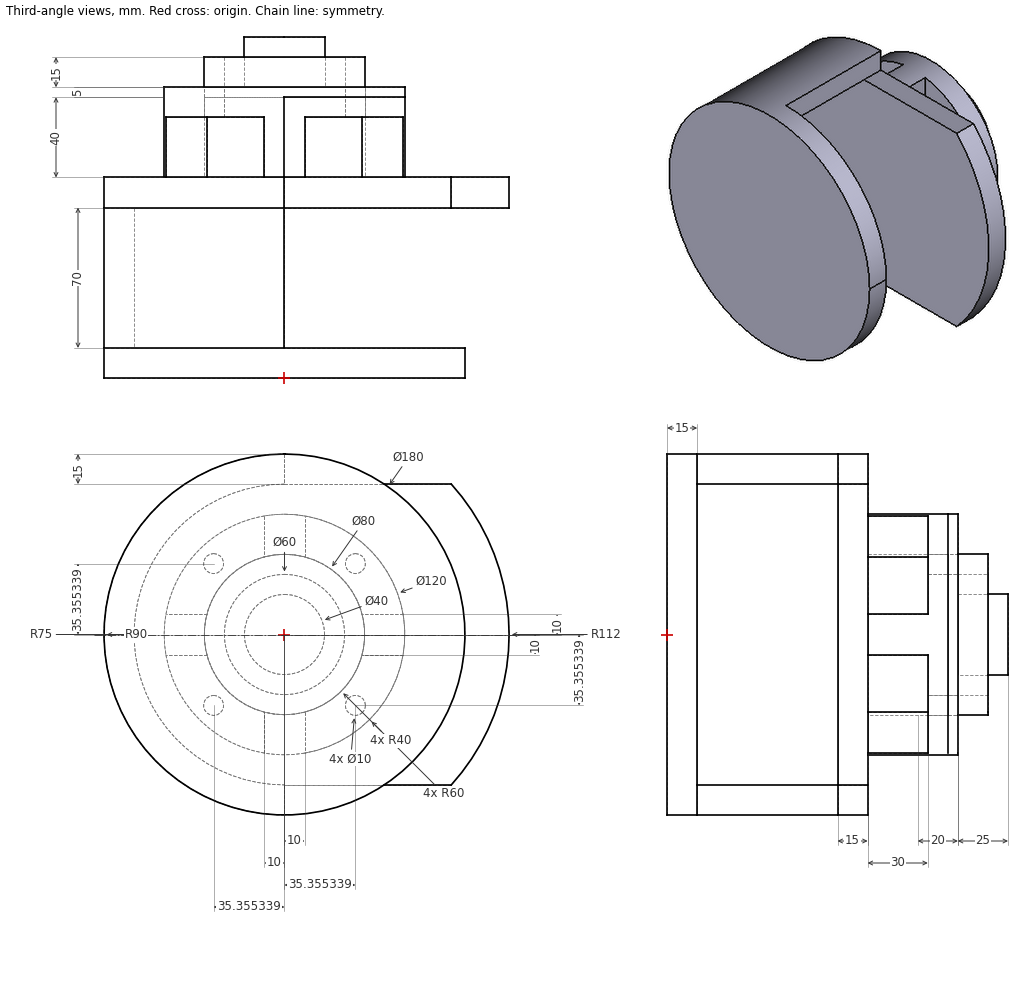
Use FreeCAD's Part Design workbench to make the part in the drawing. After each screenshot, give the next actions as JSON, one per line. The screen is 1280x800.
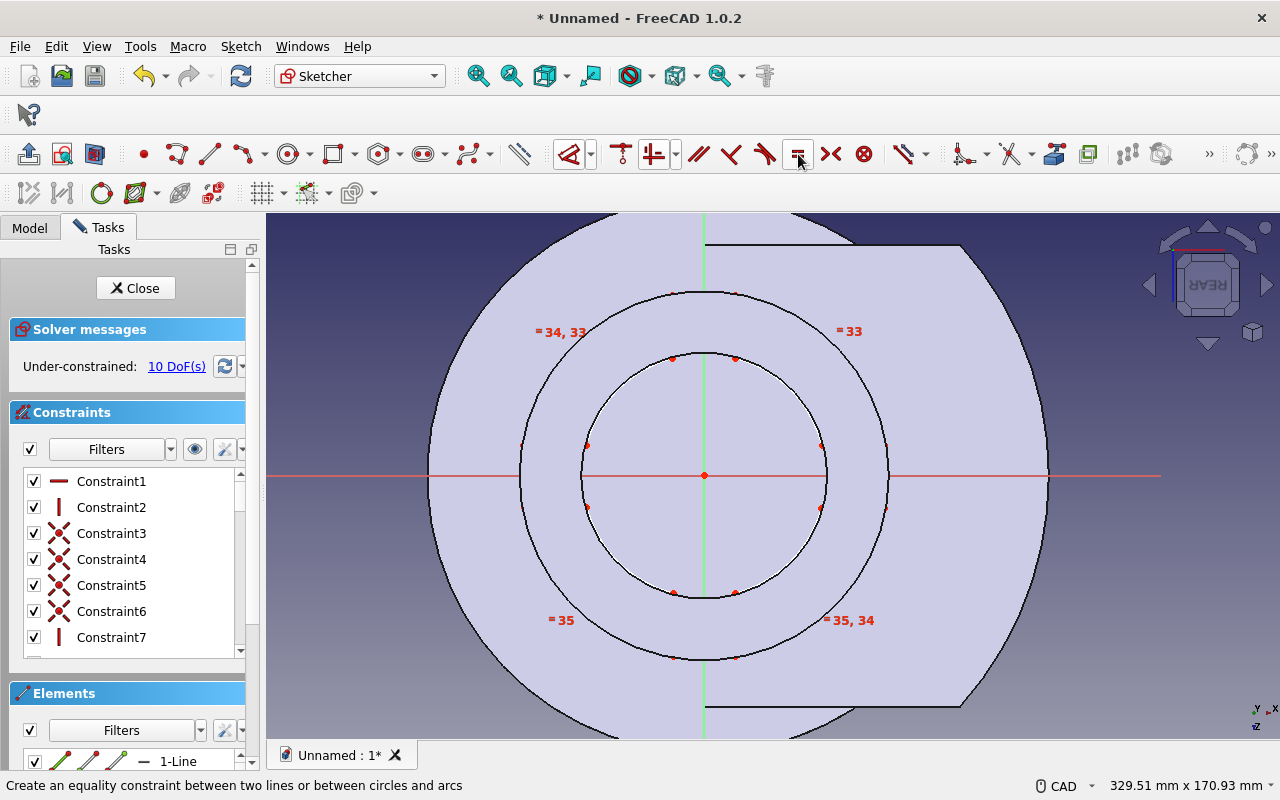
{"action": "left_click", "coordinate": [862, 382]}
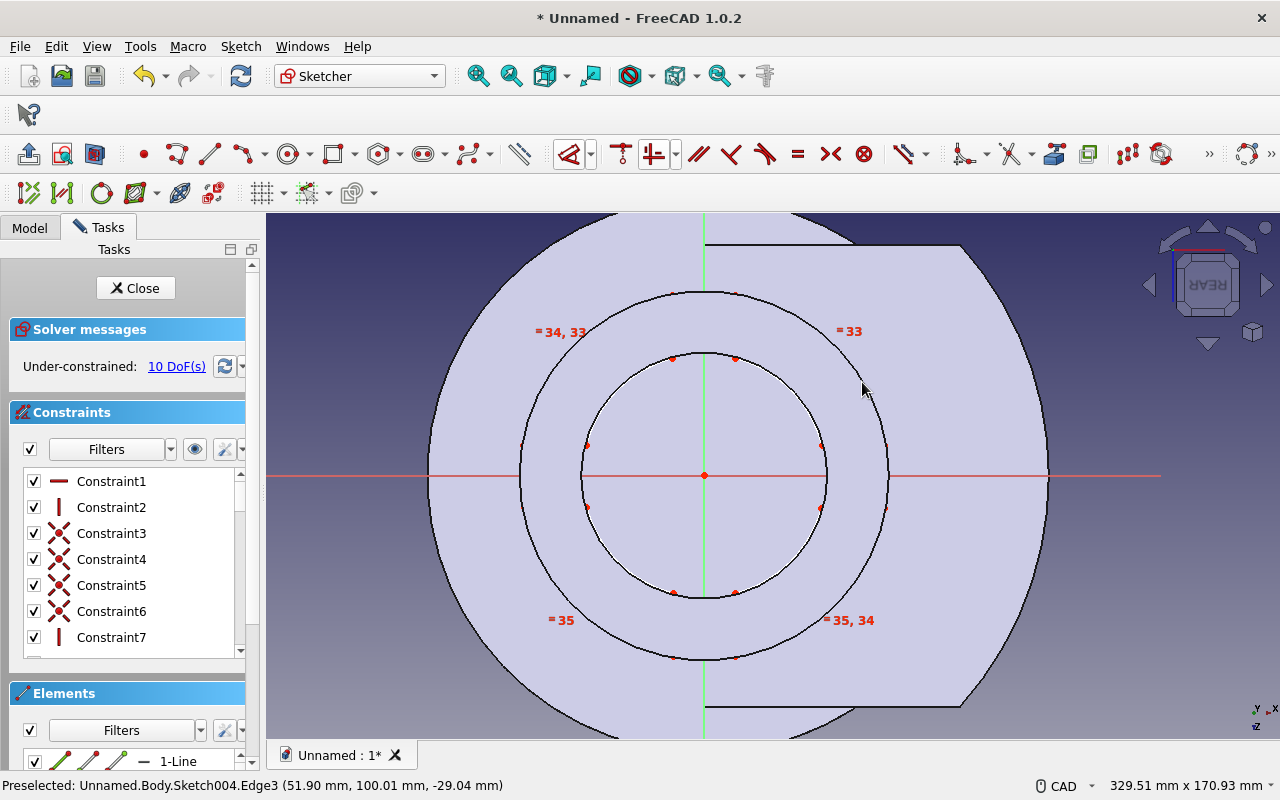
{"action": "left_click", "coordinate": [590, 154]}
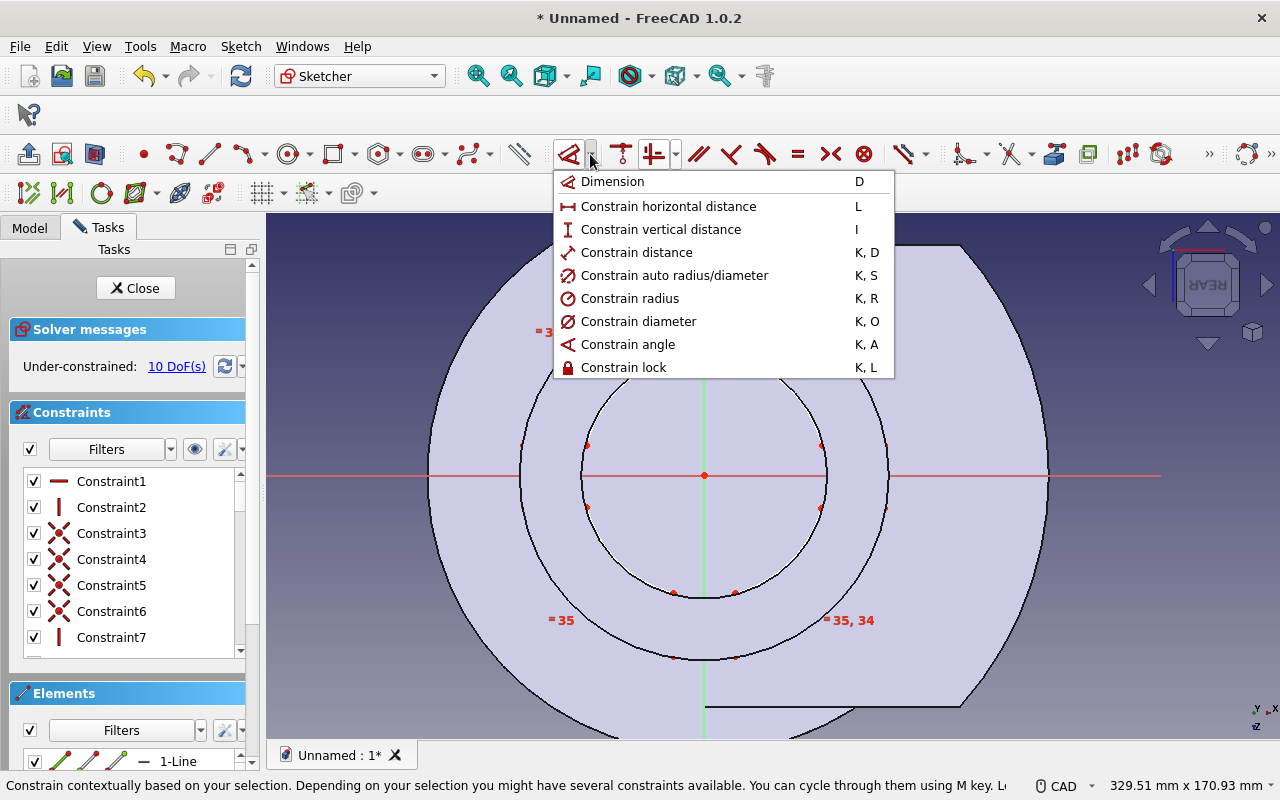
{"action": "left_click", "coordinate": [724, 298]}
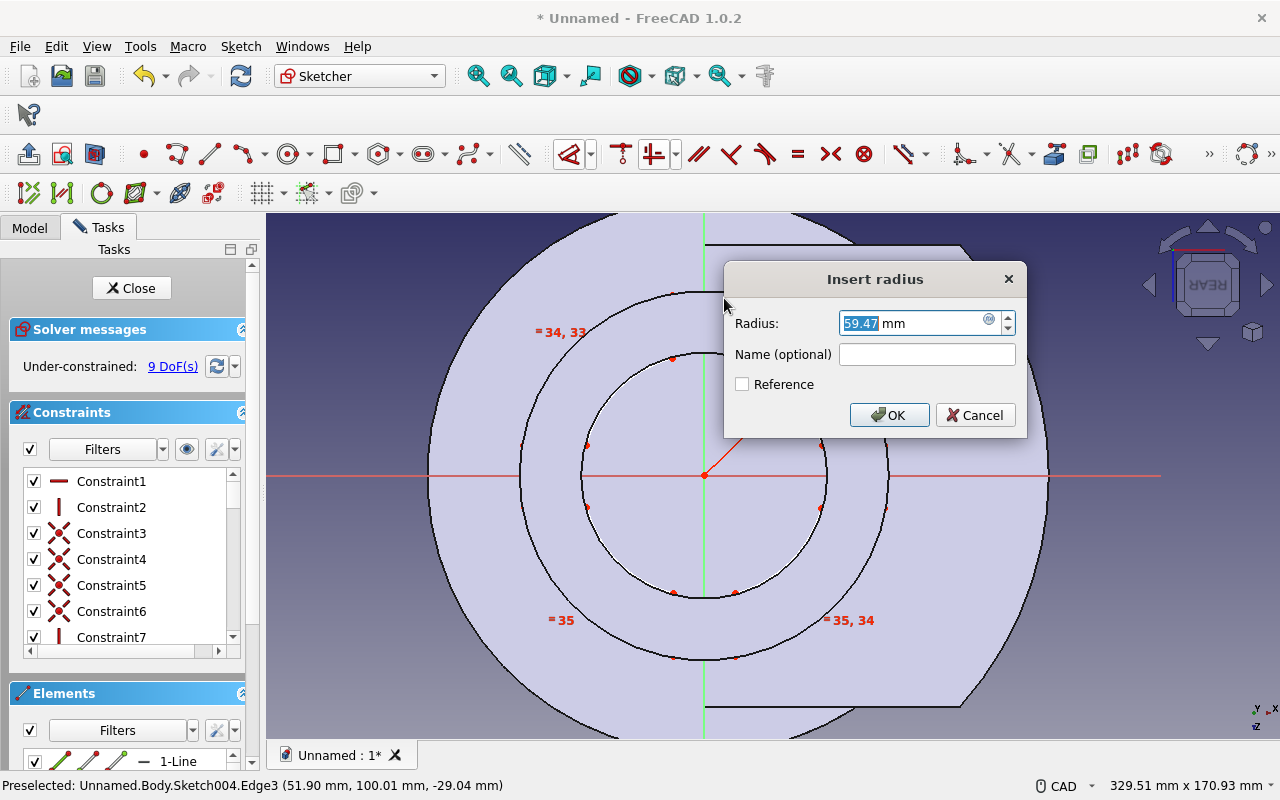
{"action": "type", "text": "60"}
{"action": "key", "text": "Return"}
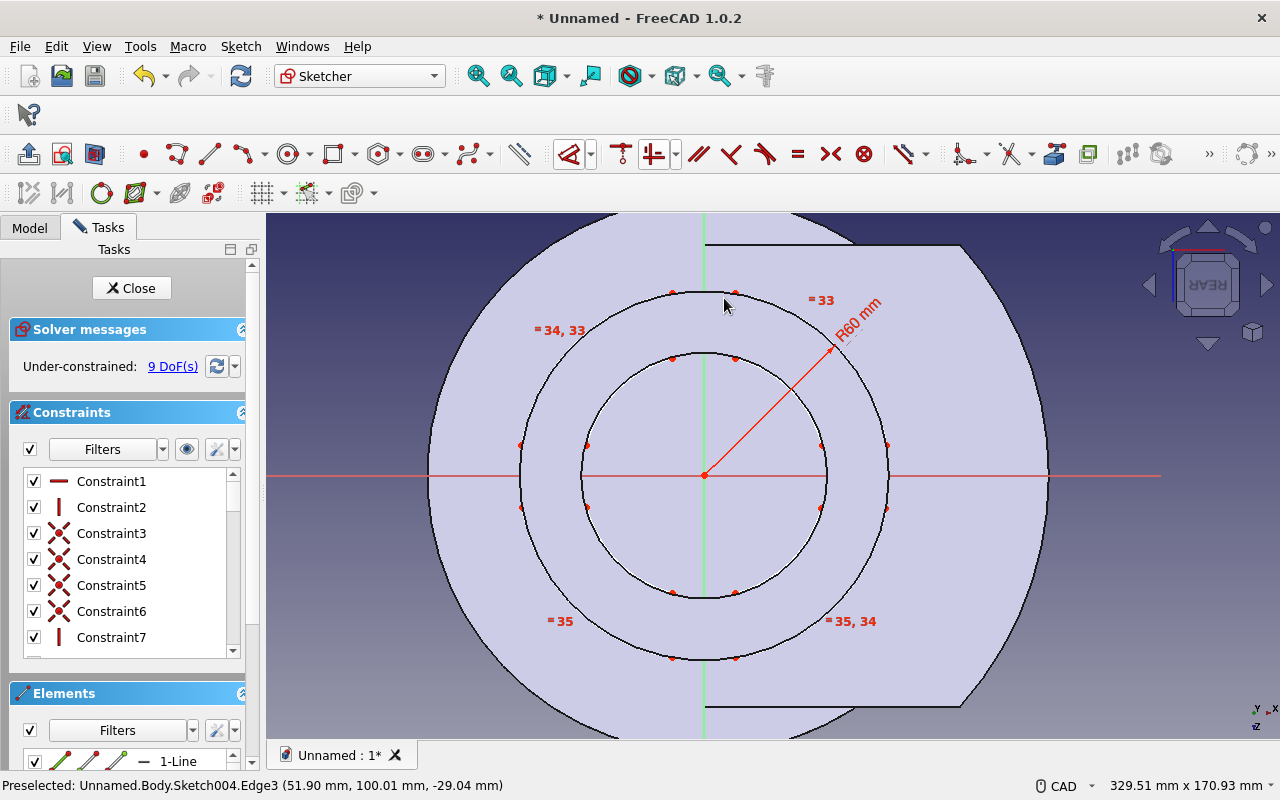
{"action": "left_click", "coordinate": [807, 410]}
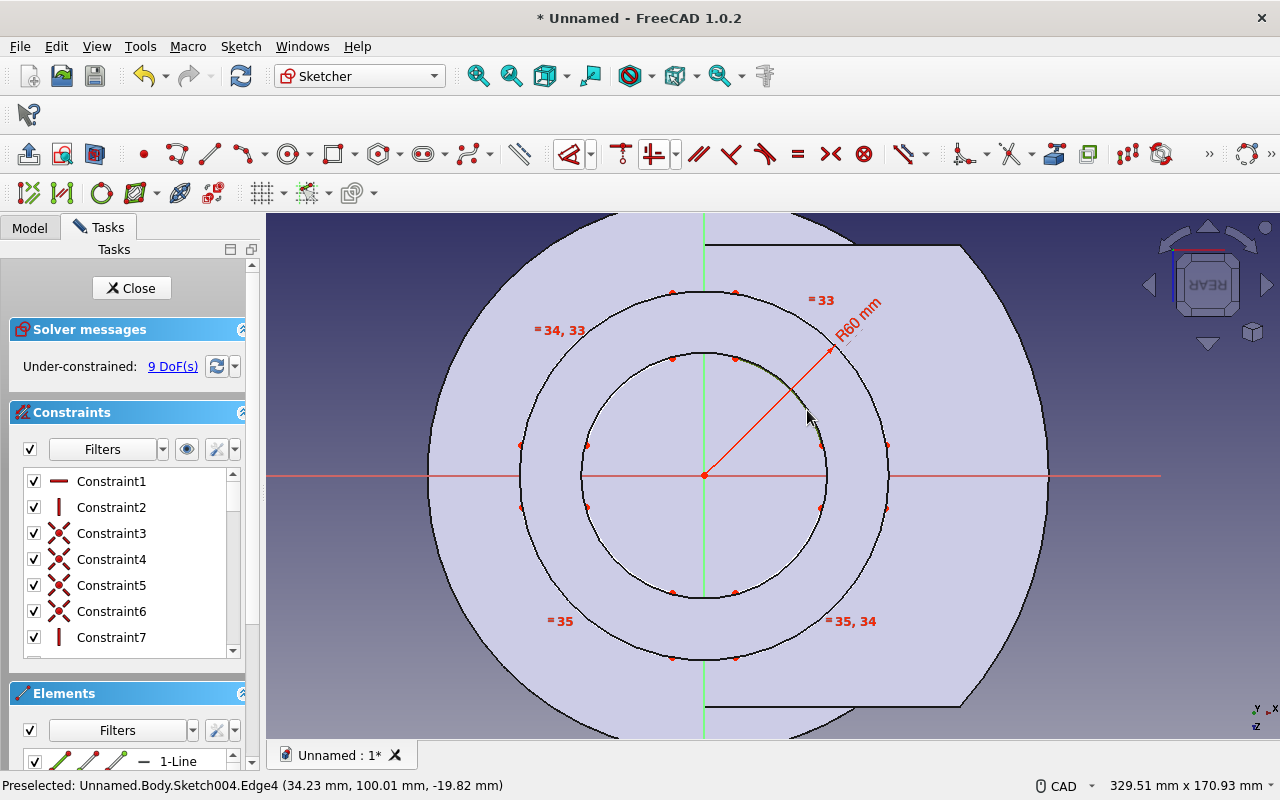
{"action": "left_click", "coordinate": [590, 154]}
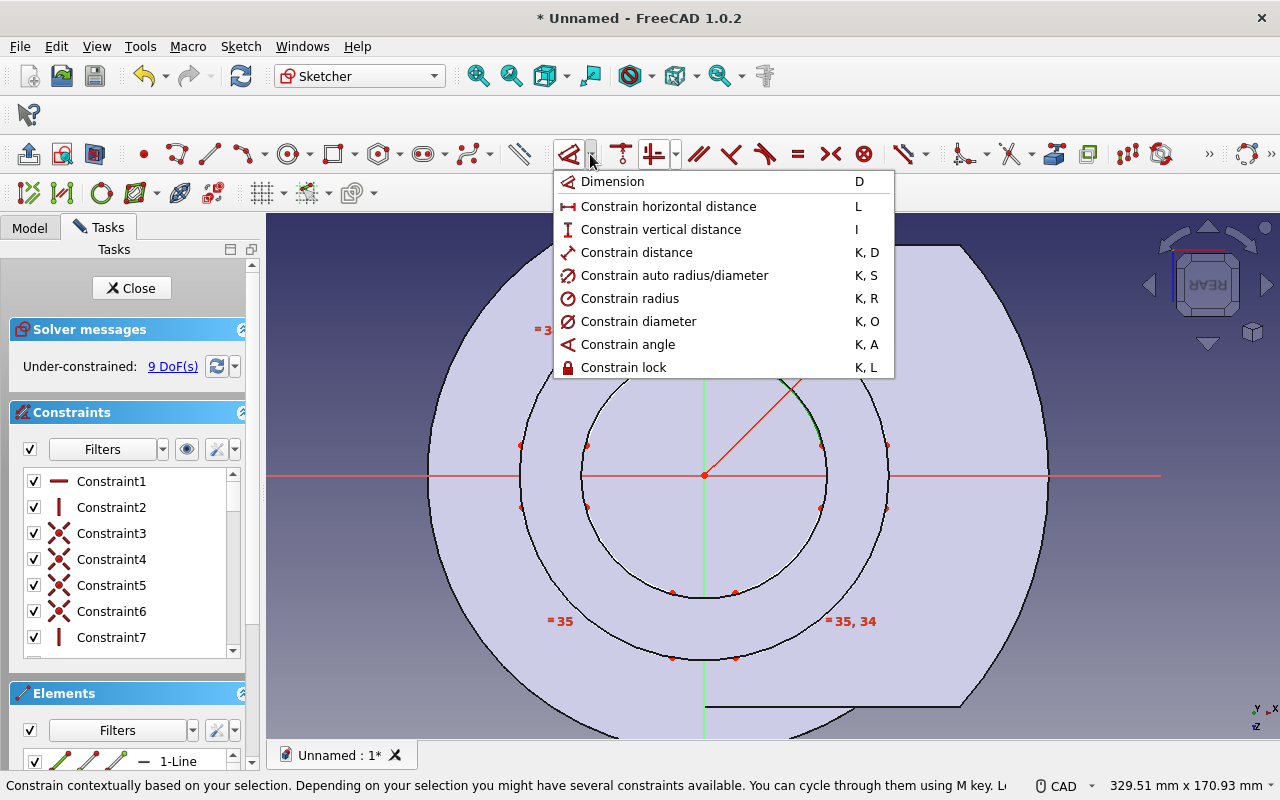
{"action": "left_click", "coordinate": [724, 298]}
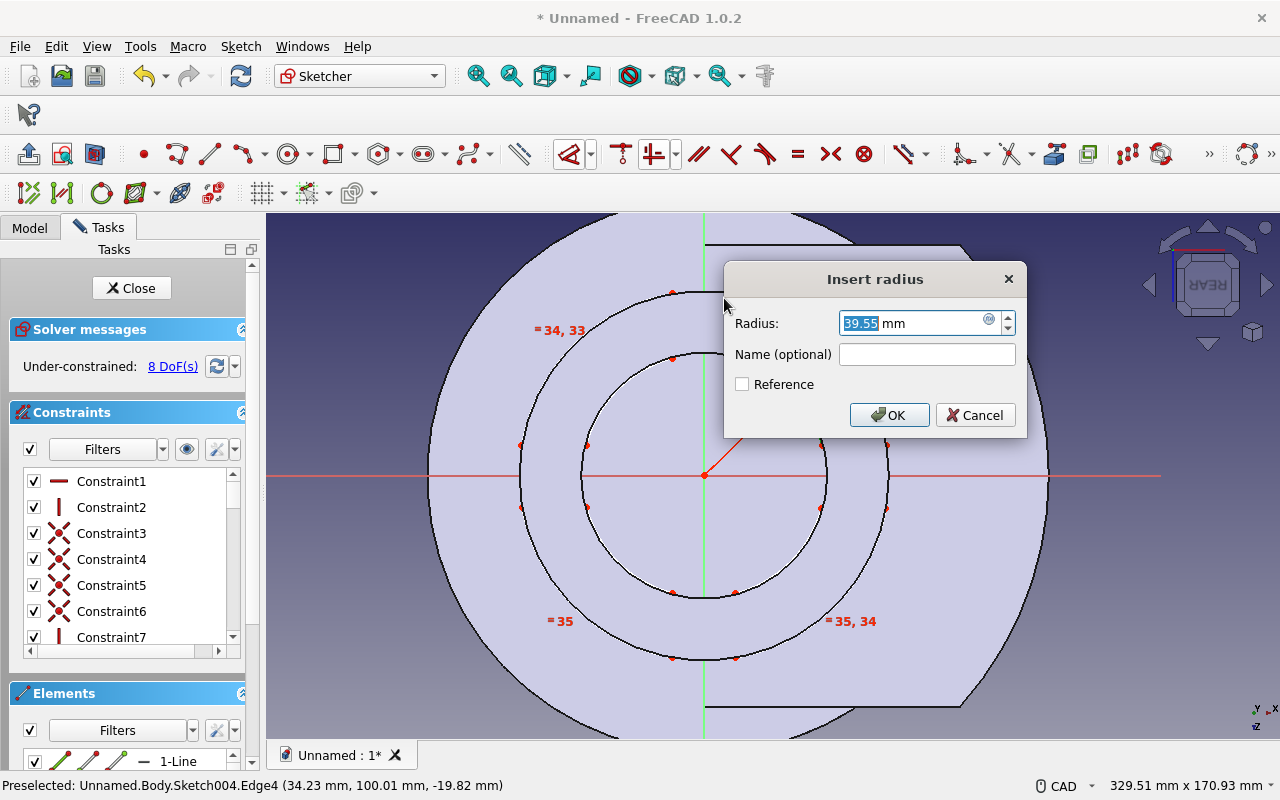
{"action": "type", "text": "40"}
{"action": "key", "text": "Return"}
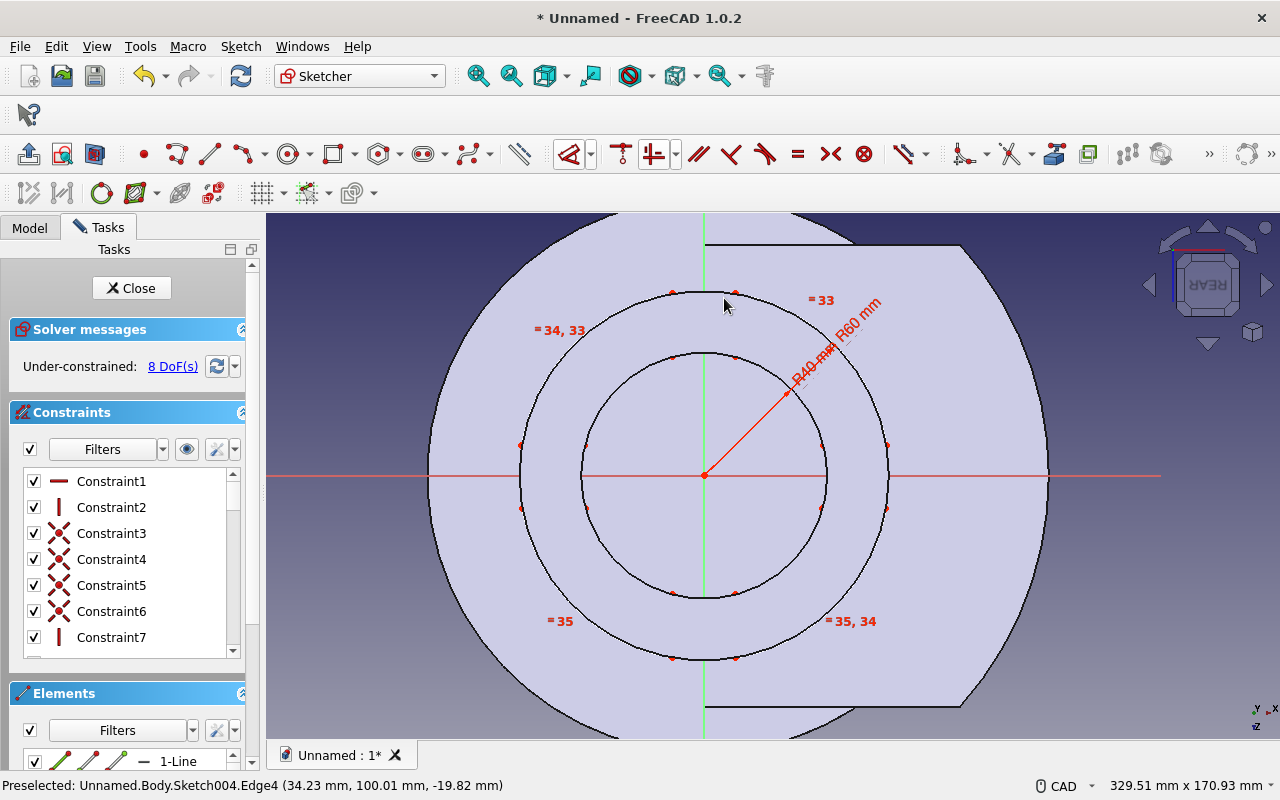
{"action": "scroll", "coordinate": [824, 446], "scroll_direction": "up", "scroll_amount": 2}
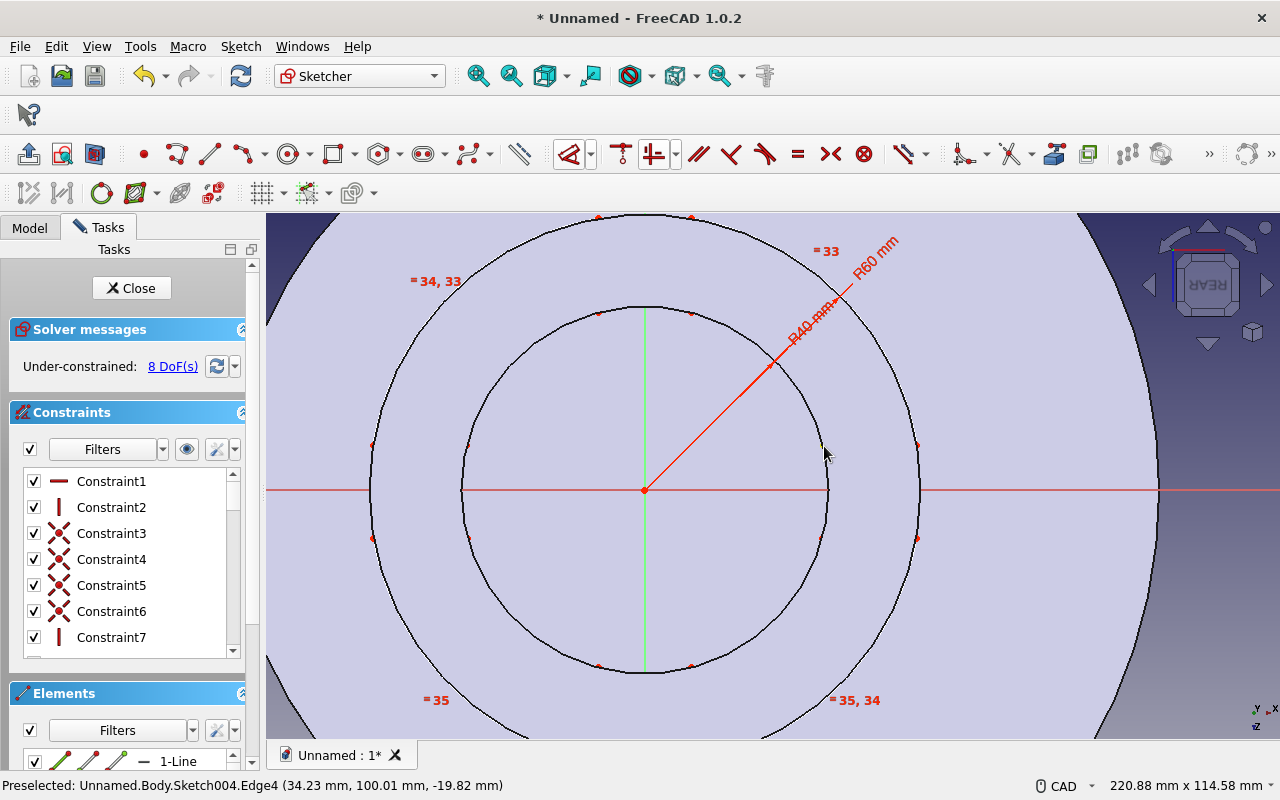
{"action": "left_click", "coordinate": [823, 446]}